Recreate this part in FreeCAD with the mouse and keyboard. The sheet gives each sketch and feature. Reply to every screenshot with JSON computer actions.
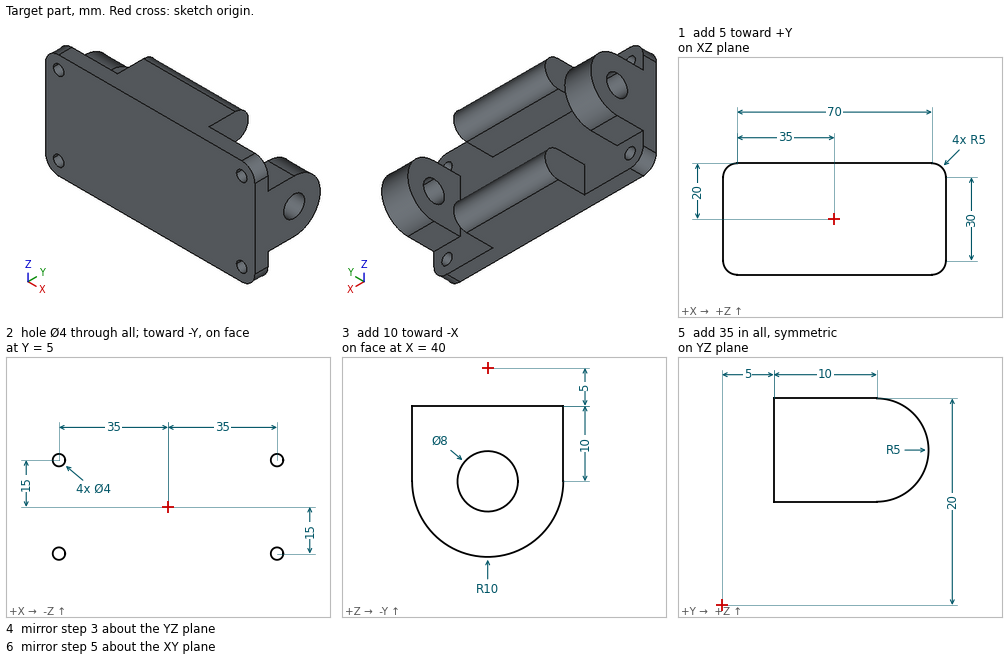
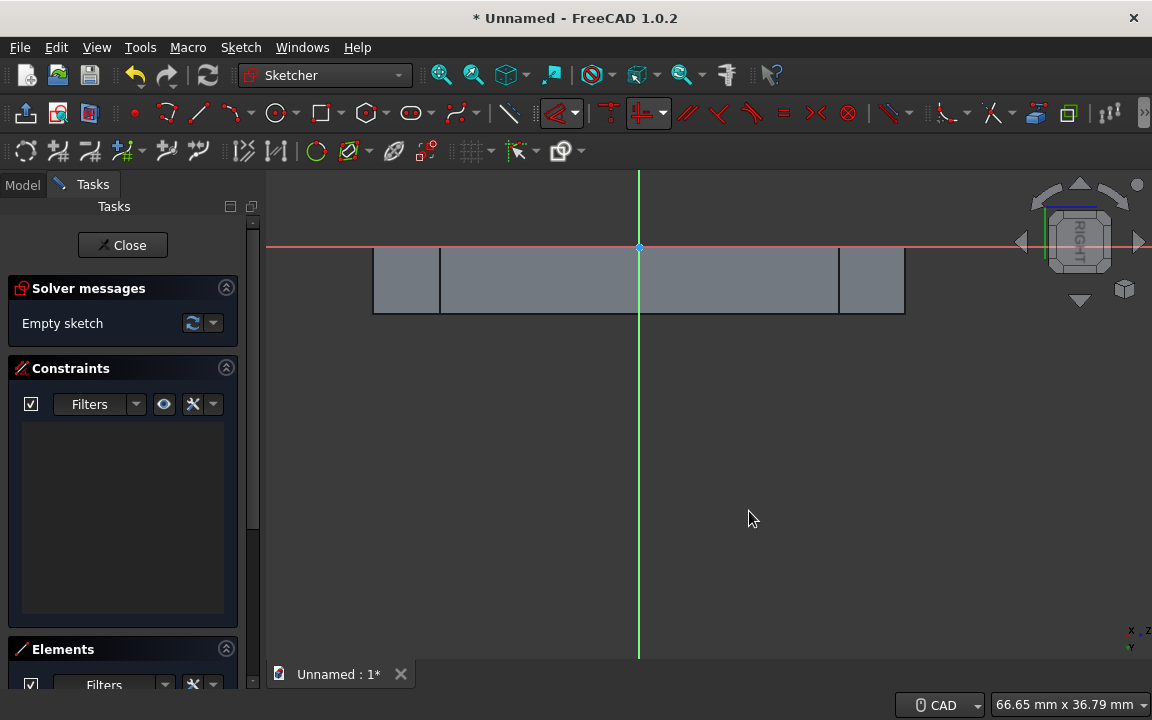
{"action": "left_click", "coordinate": [168, 114]}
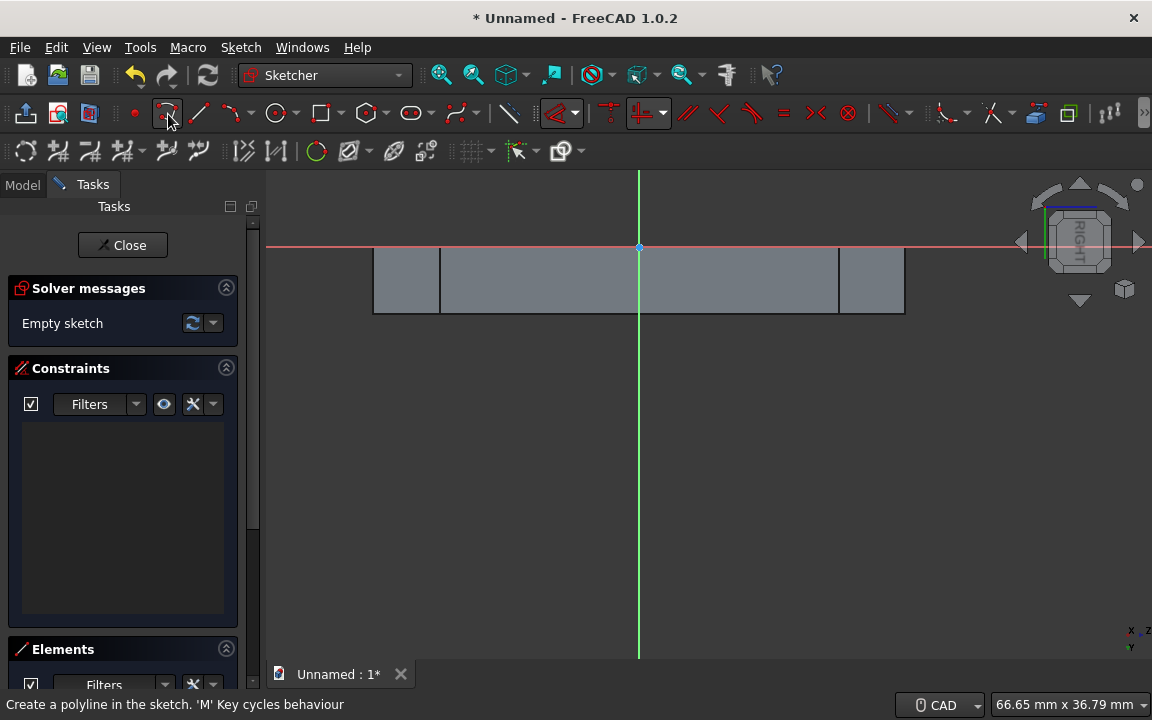
{"action": "left_click", "coordinate": [772, 447]}
{"action": "left_click", "coordinate": [772, 314]}
{"action": "left_click", "coordinate": [506, 314]}
{"action": "left_click", "coordinate": [506, 447]}
{"action": "right_click", "coordinate": [506, 447]}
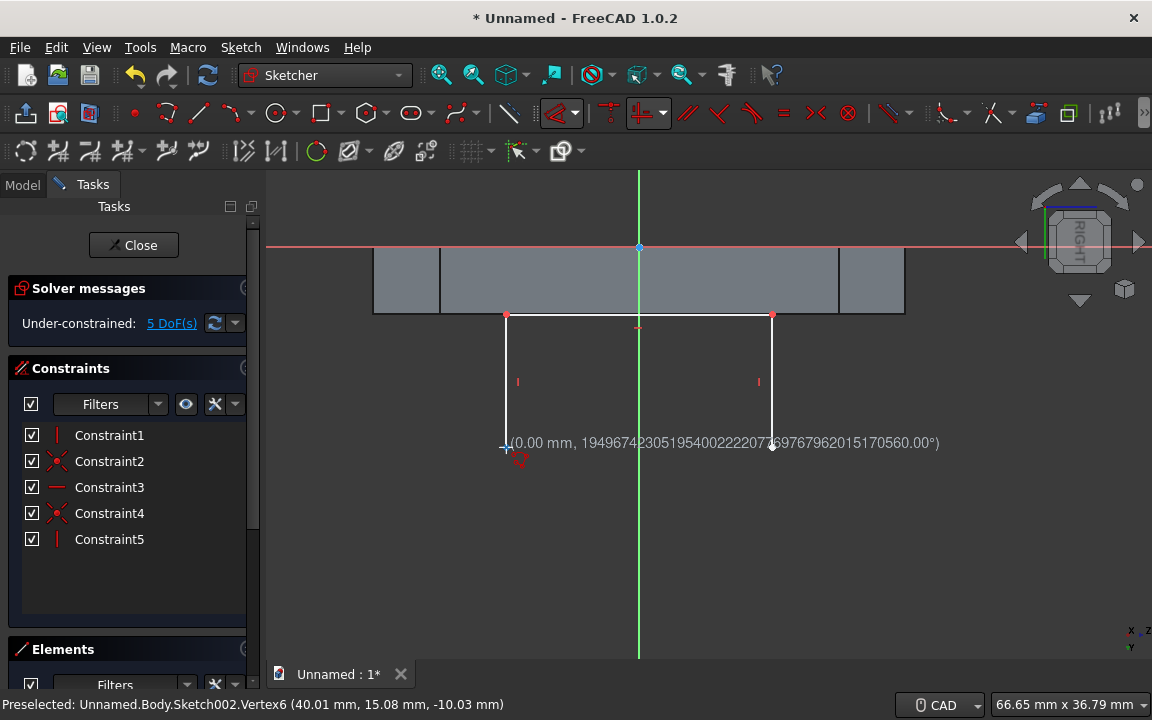
{"action": "left_click", "coordinate": [232, 114]}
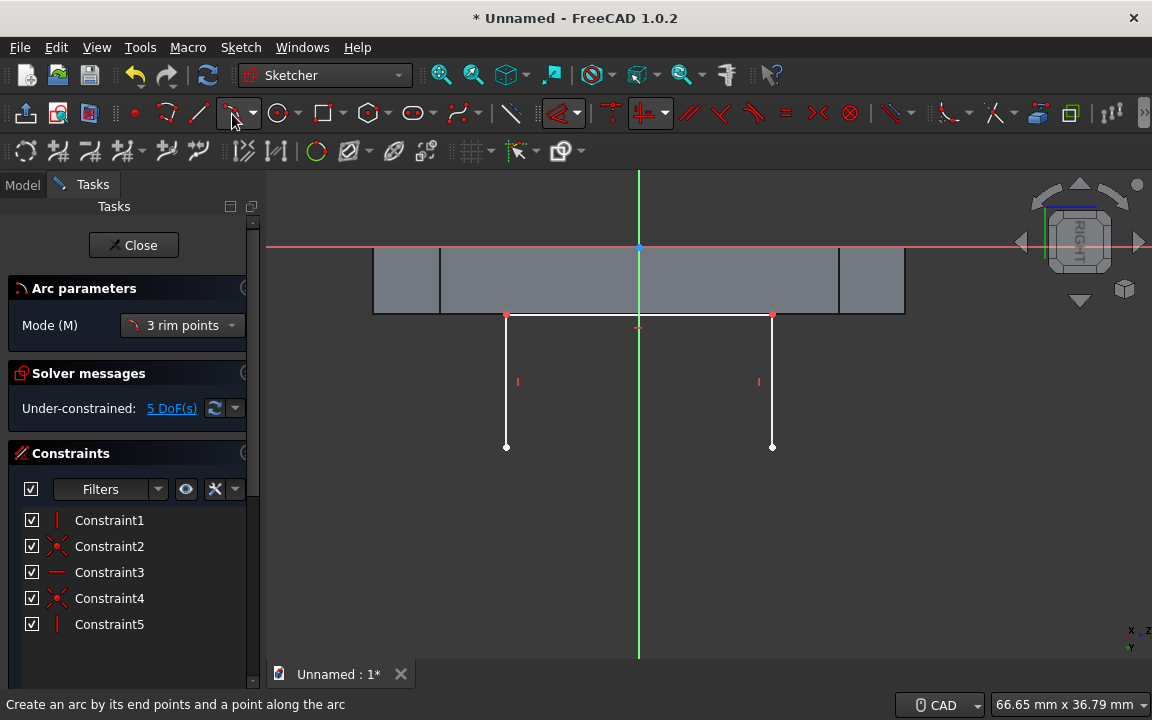
{"action": "left_click", "coordinate": [506, 448]}
{"action": "left_click", "coordinate": [772, 448]}
{"action": "left_click", "coordinate": [598, 573]}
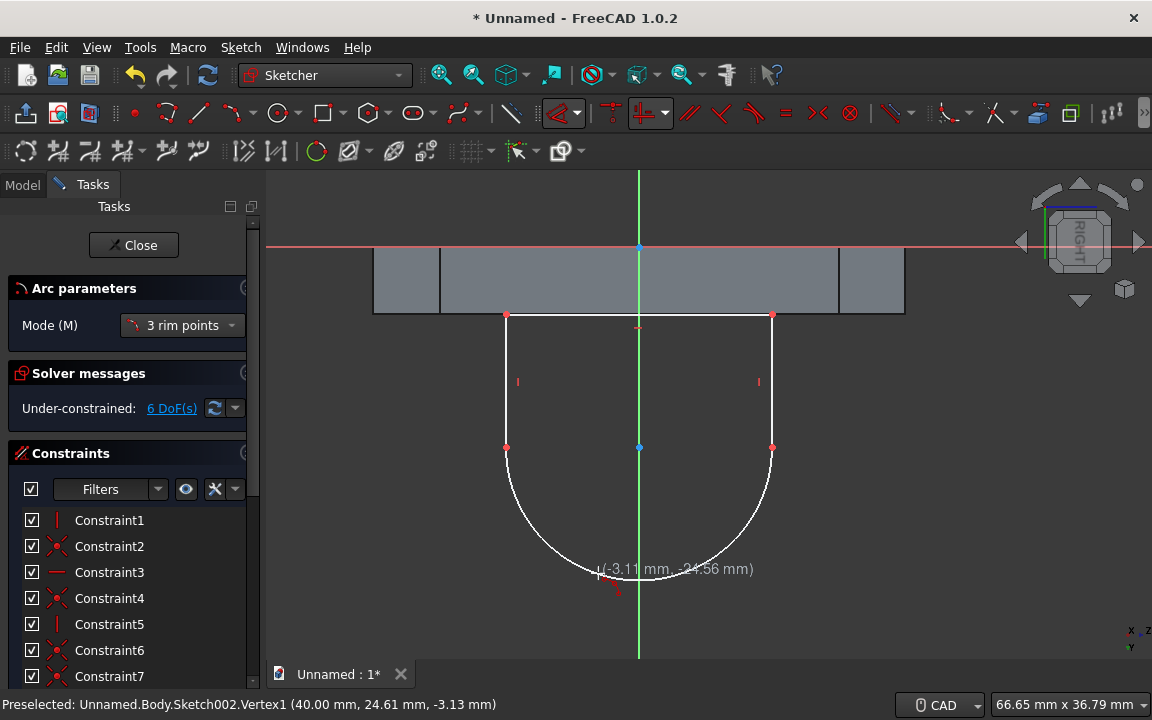
{"action": "key", "text": "g c"}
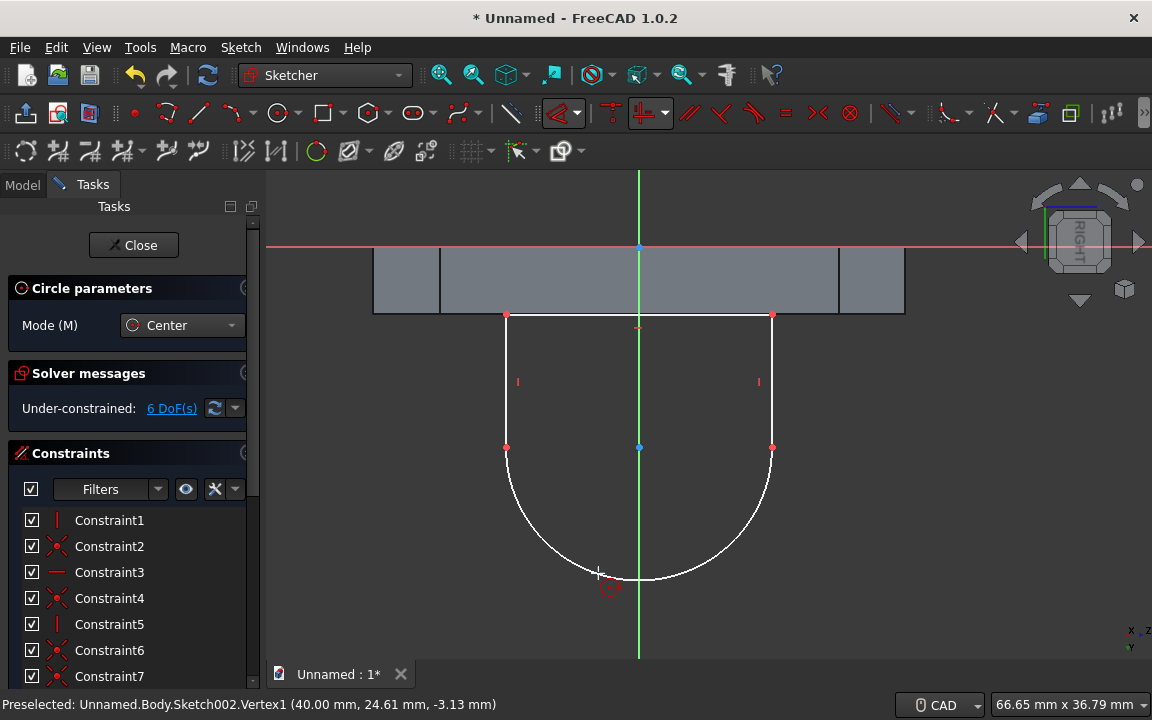
{"action": "left_click", "coordinate": [639, 447]}
{"action": "left_click", "coordinate": [677, 409]}
{"action": "key", "text": "Escape"}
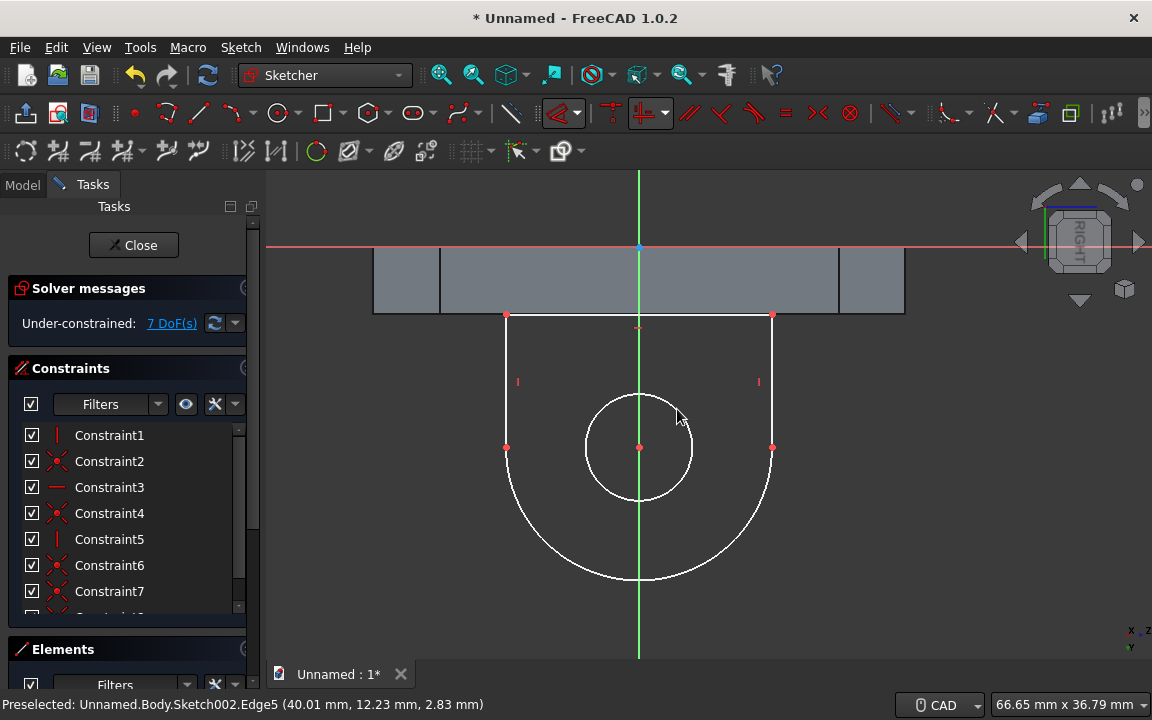
{"action": "left_click", "coordinate": [772, 408]}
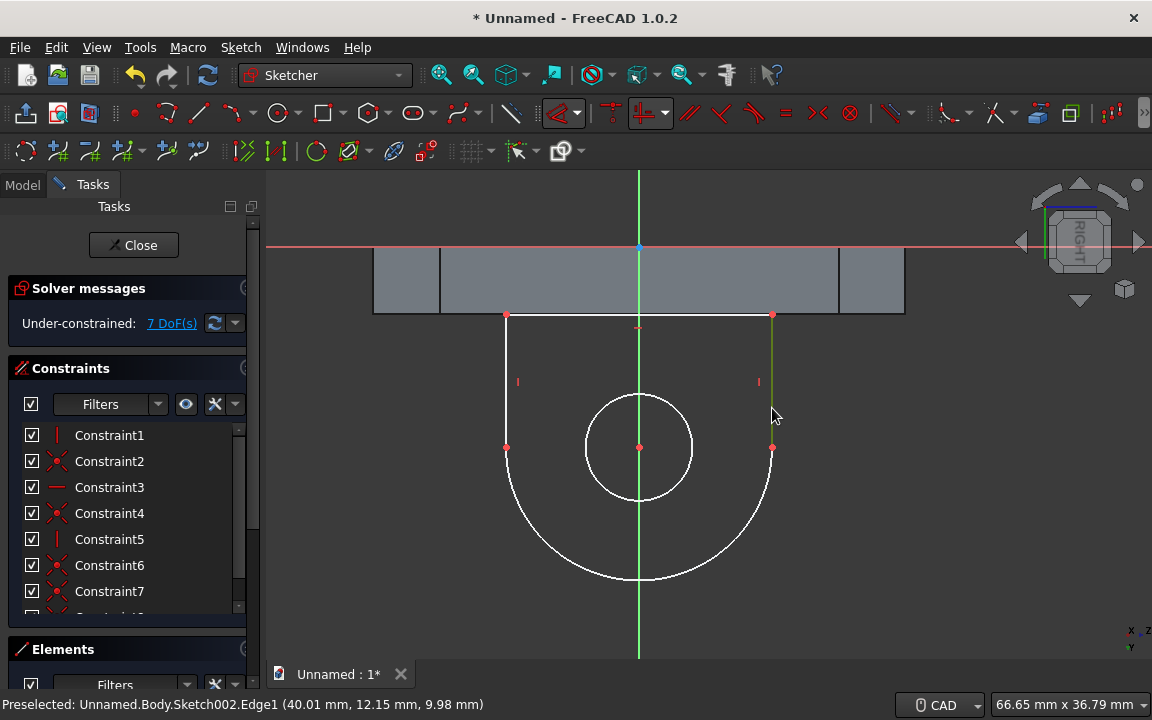
{"action": "left_click", "coordinate": [561, 555]}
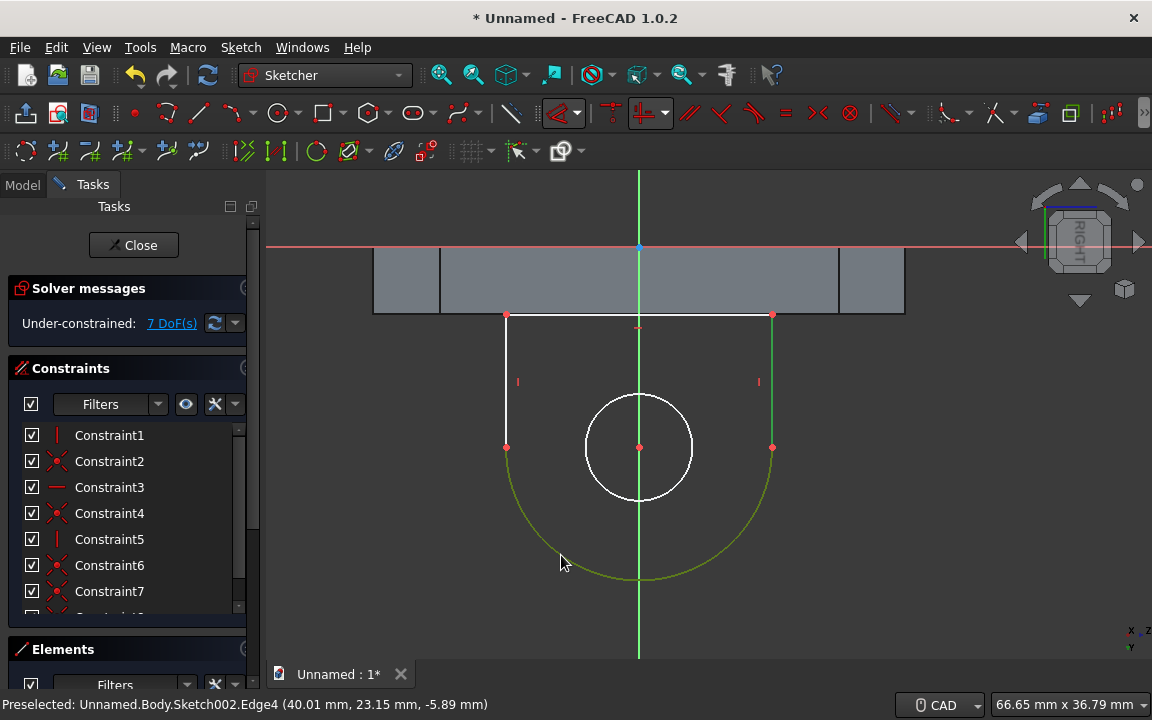
{"action": "left_click", "coordinate": [754, 114]}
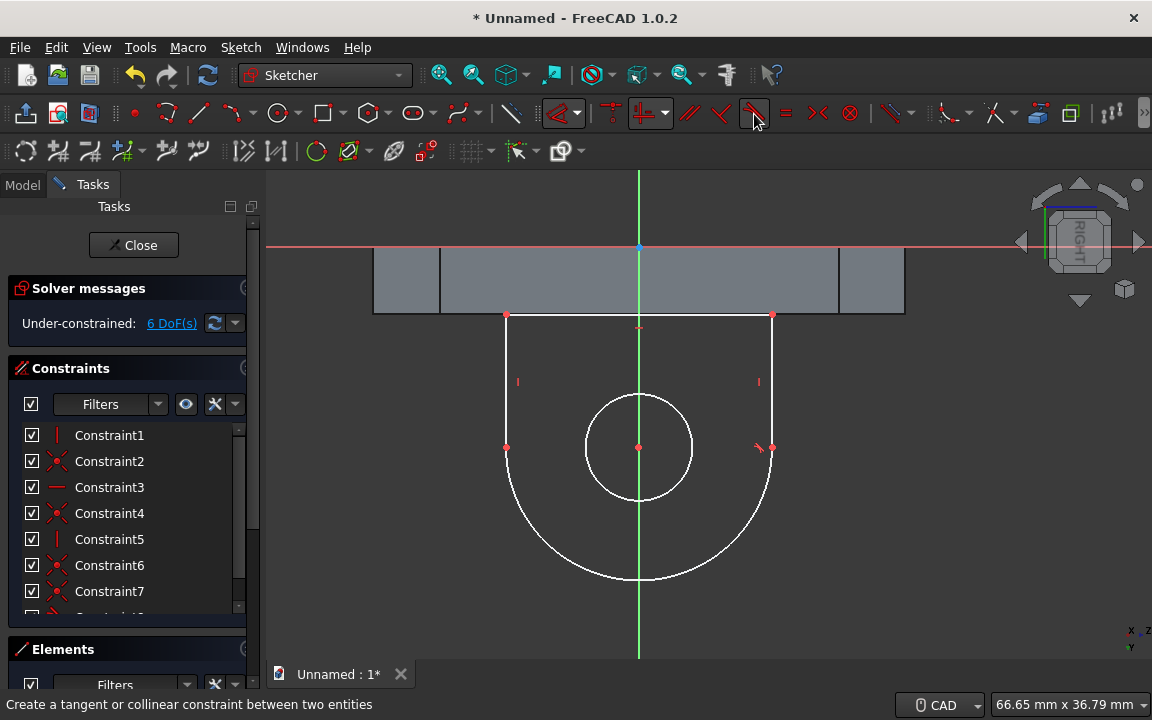
{"action": "left_click", "coordinate": [506, 355]}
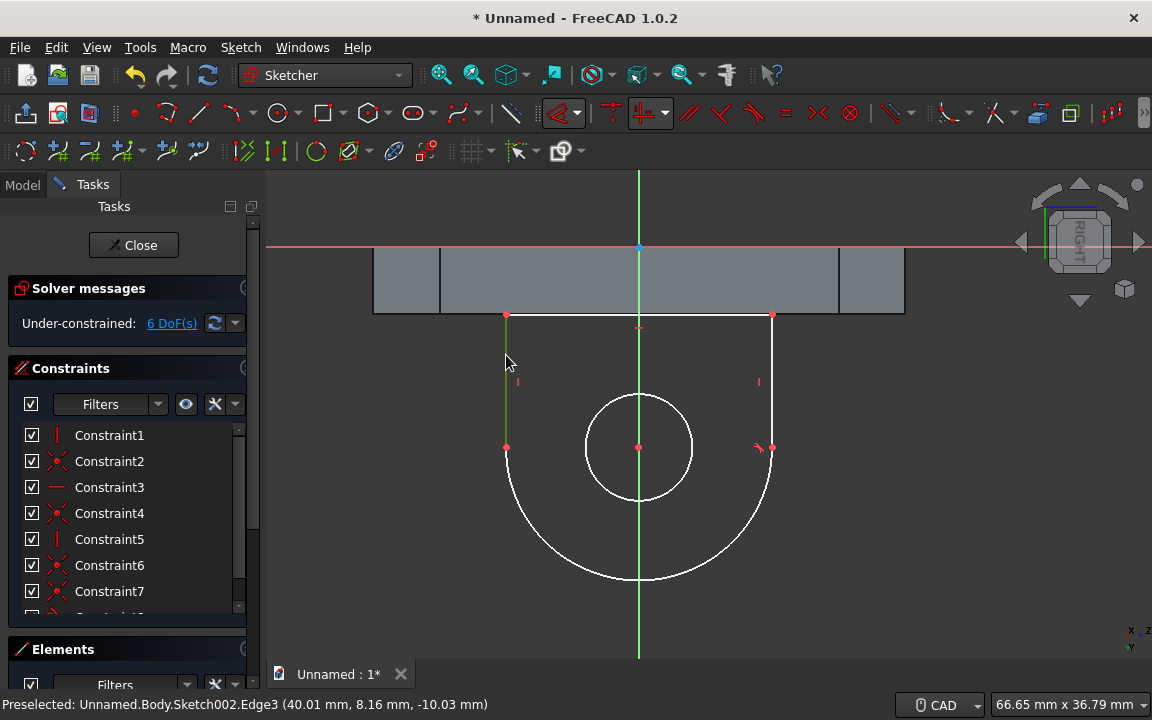
{"action": "left_click", "coordinate": [561, 555]}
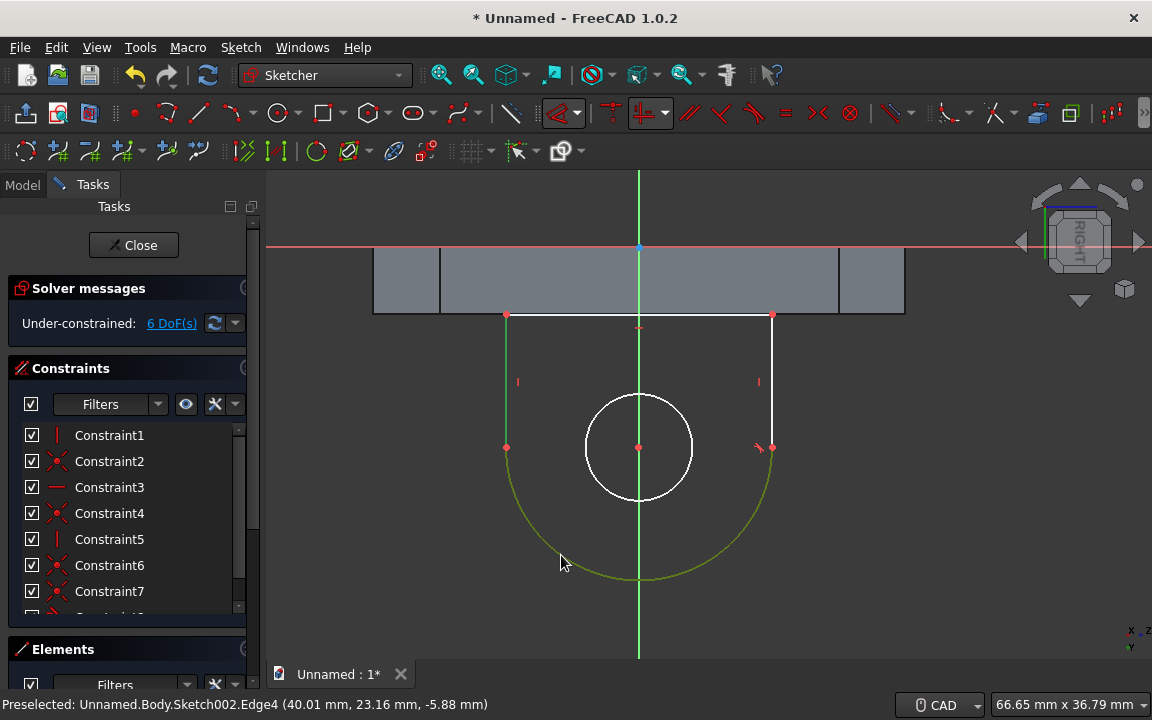
{"action": "key", "text": "t"}